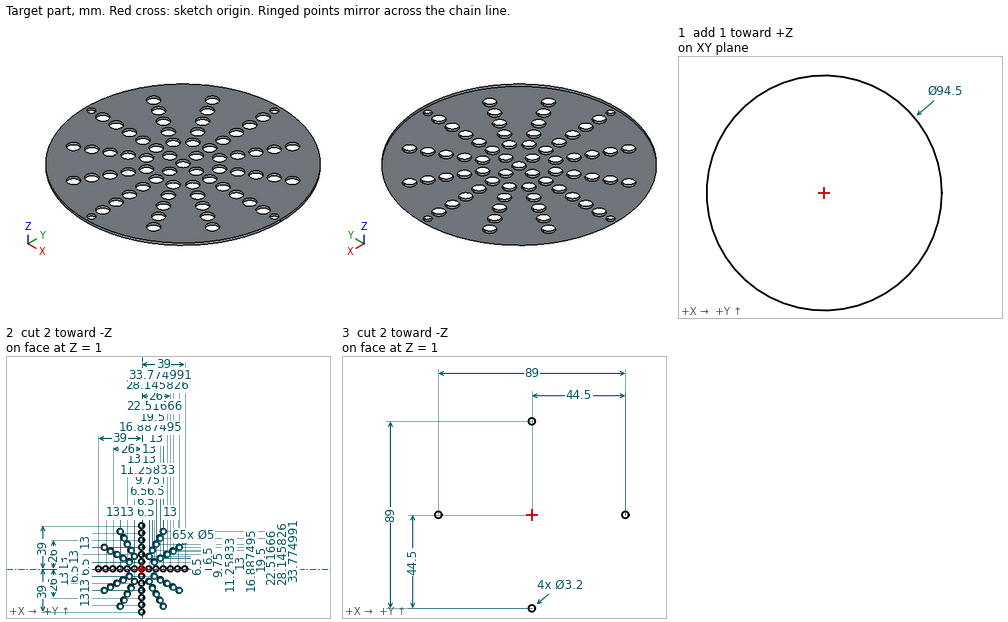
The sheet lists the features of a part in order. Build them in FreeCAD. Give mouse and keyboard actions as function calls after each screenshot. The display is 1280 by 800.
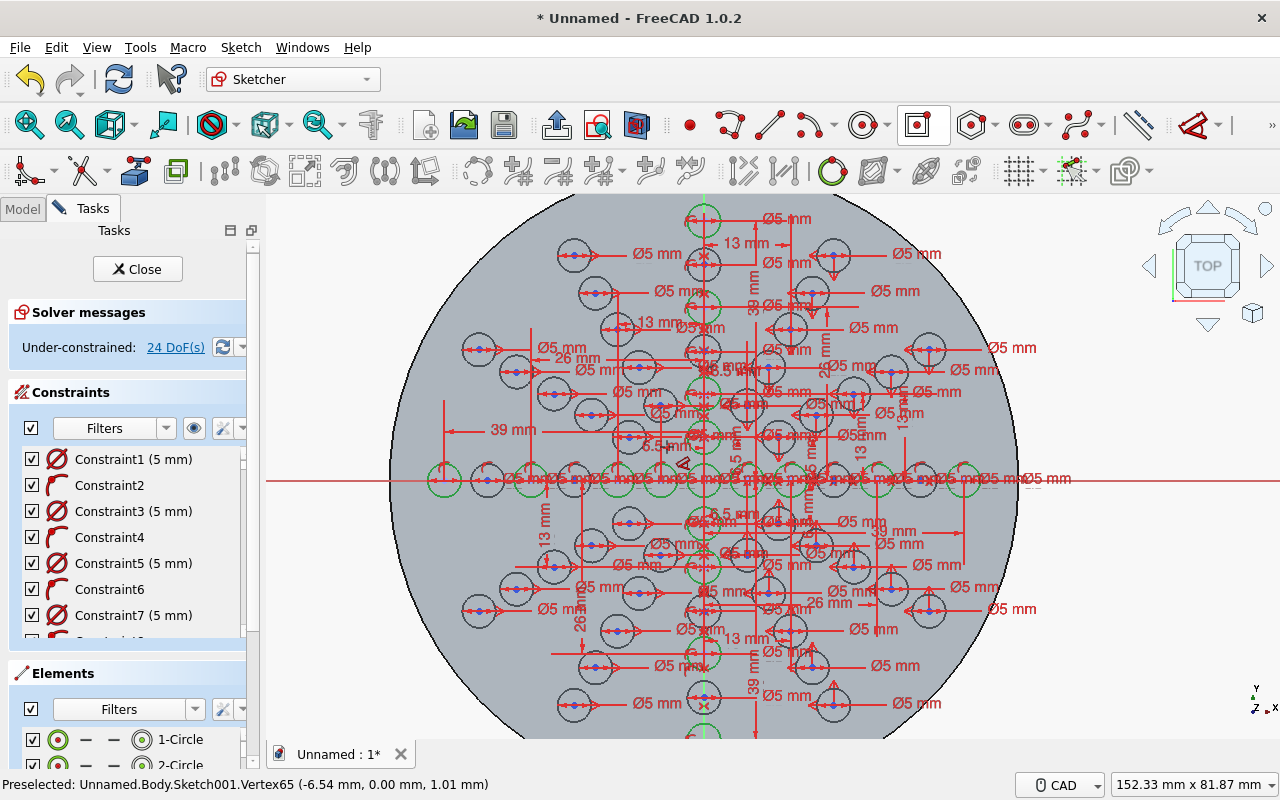
click(704, 437)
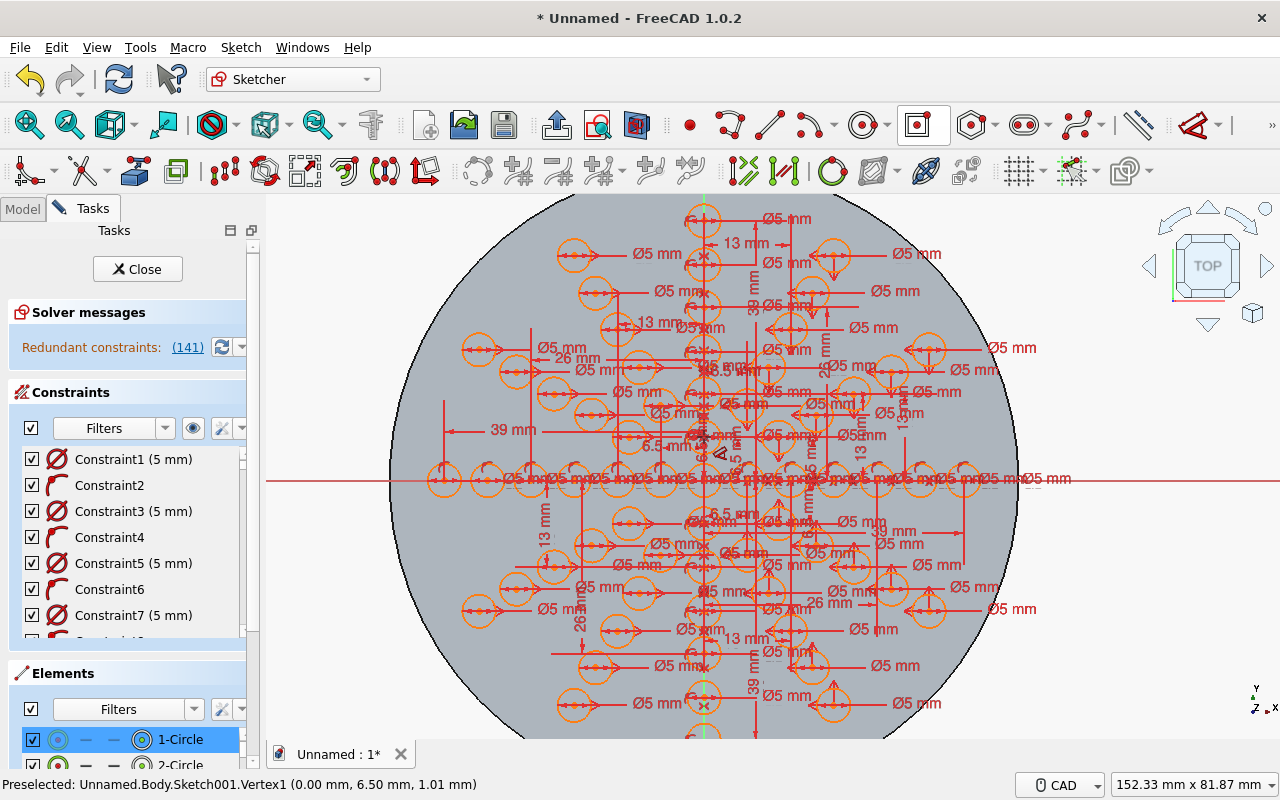
click(704, 352)
click(786, 394)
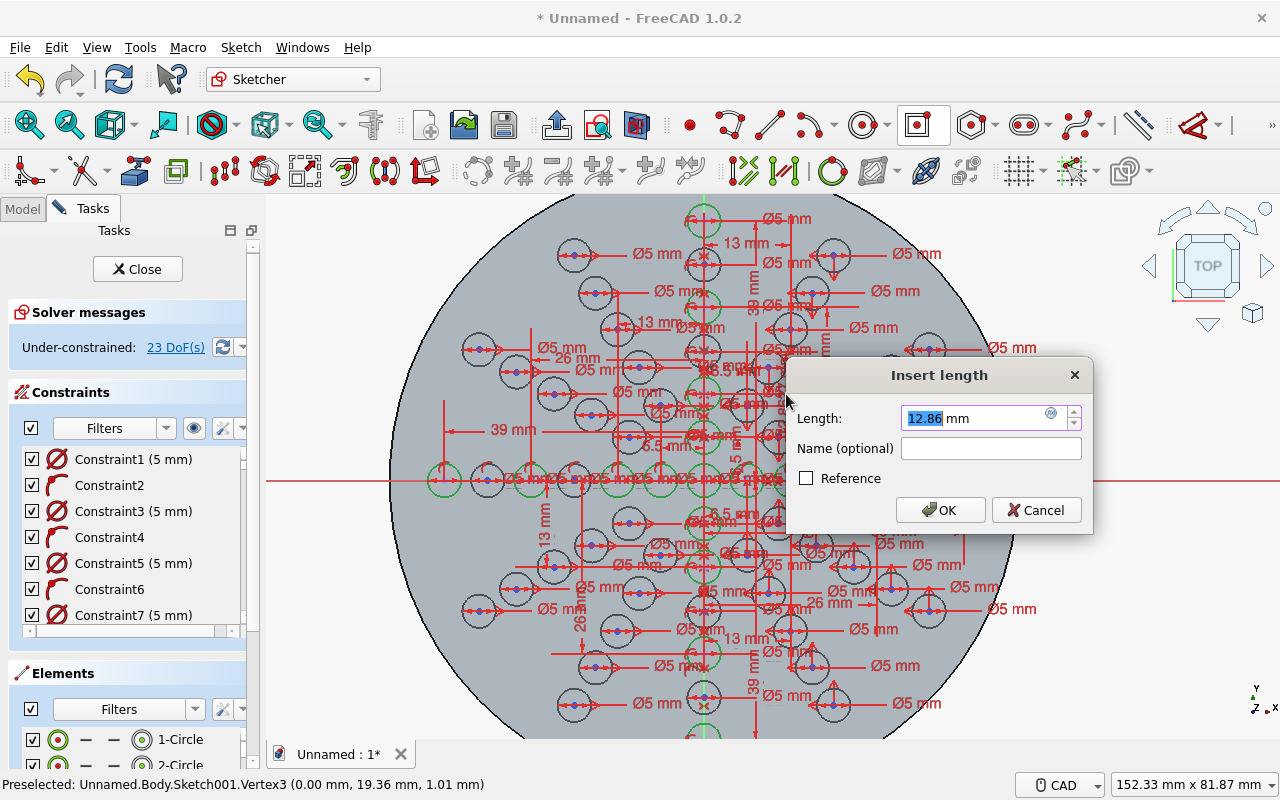
text(13)
key(Return)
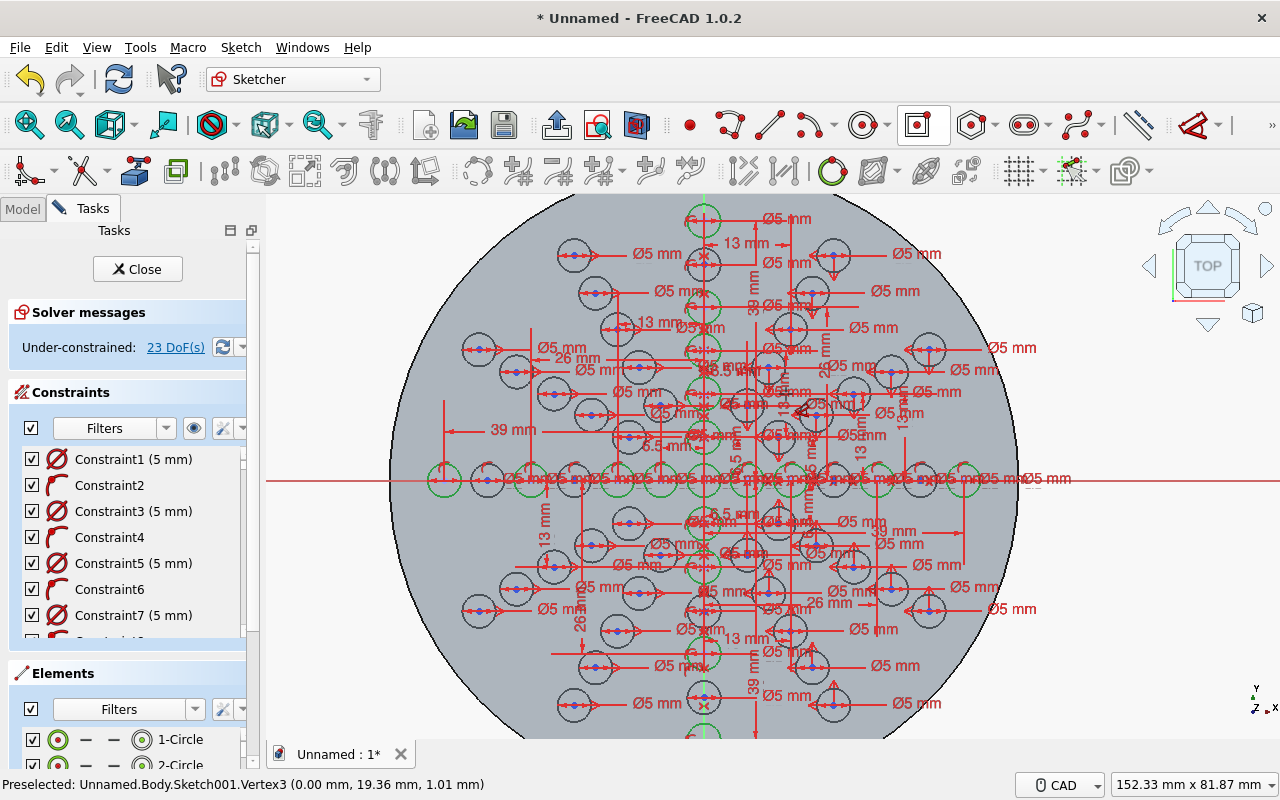
click(704, 351)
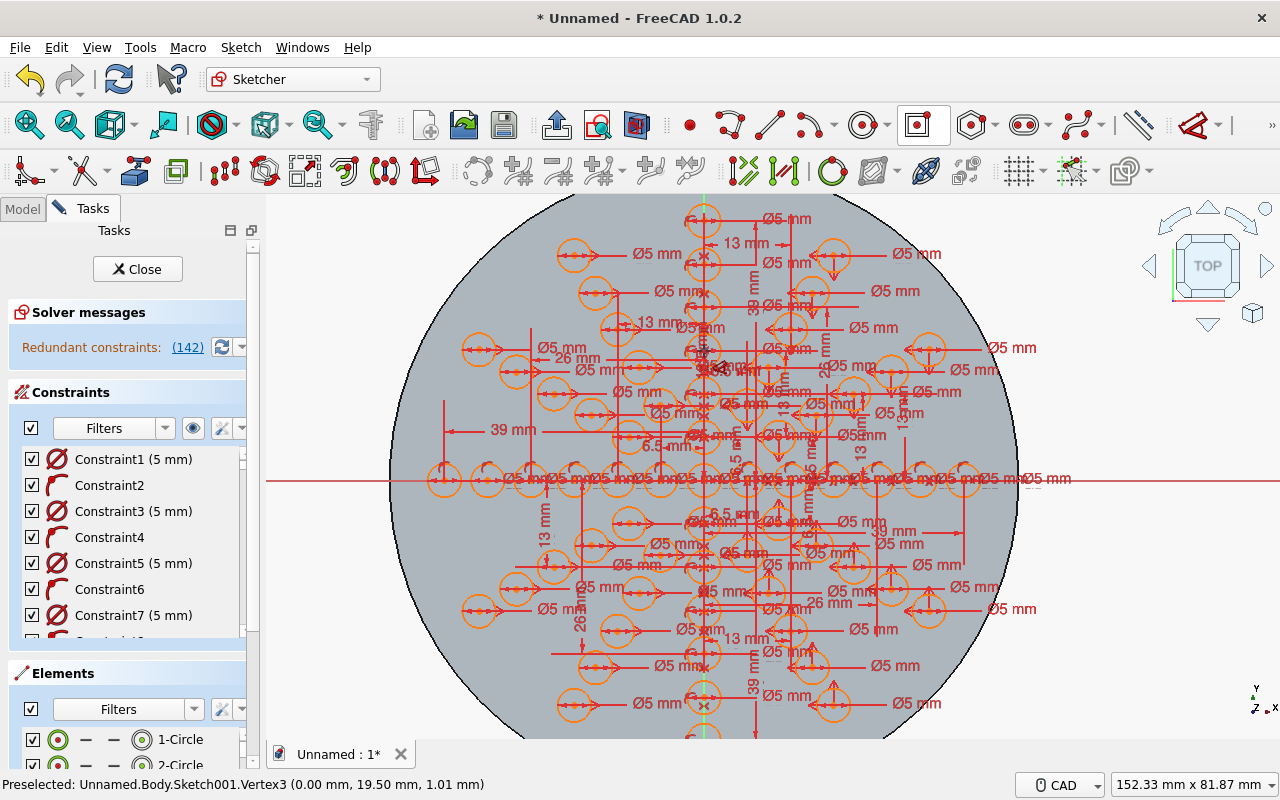
click(704, 265)
click(738, 328)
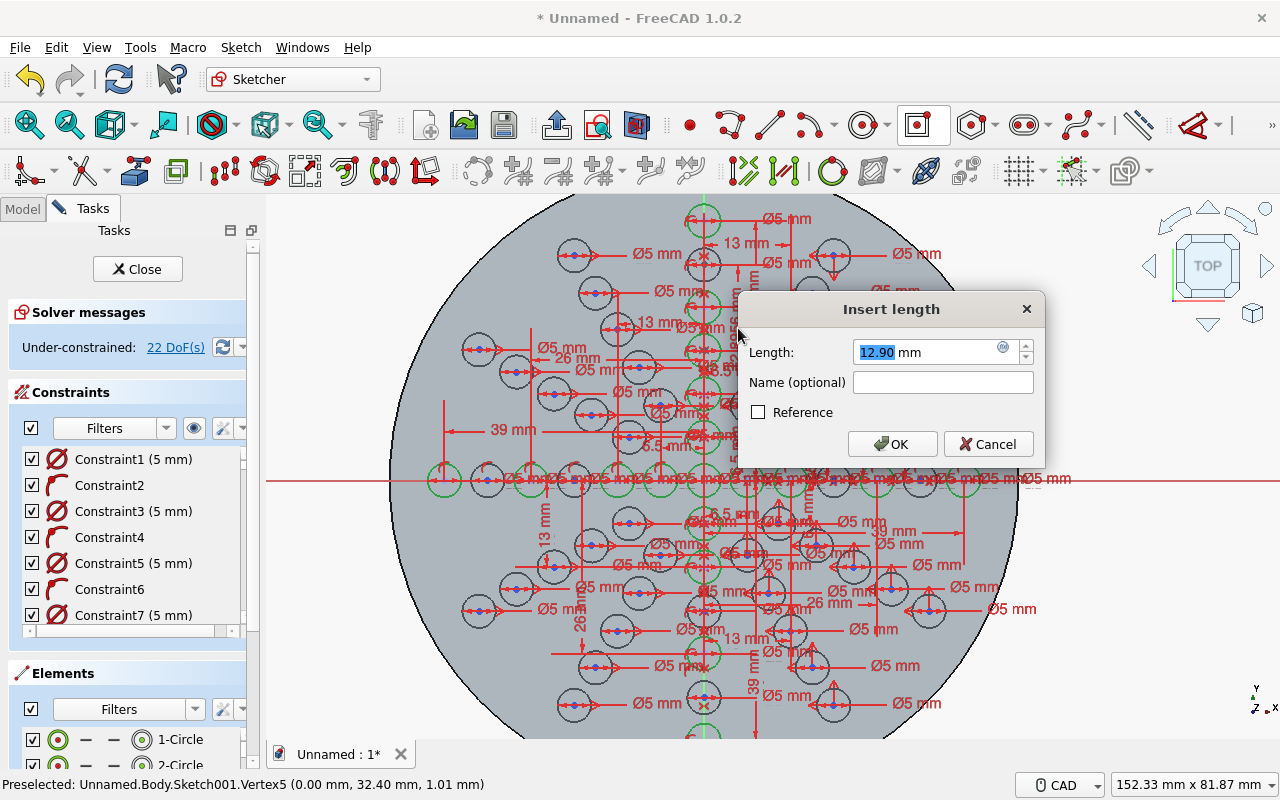
text(13)
key(Return)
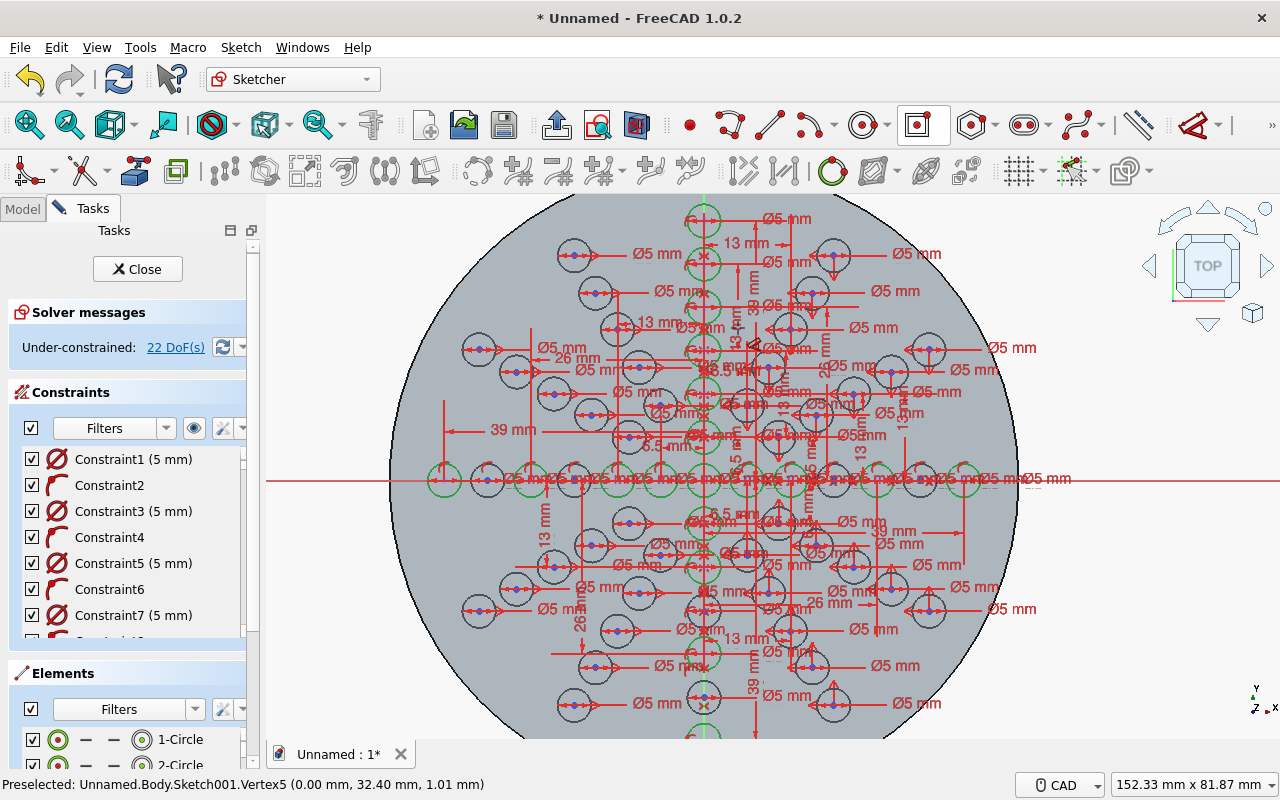
click(920, 481)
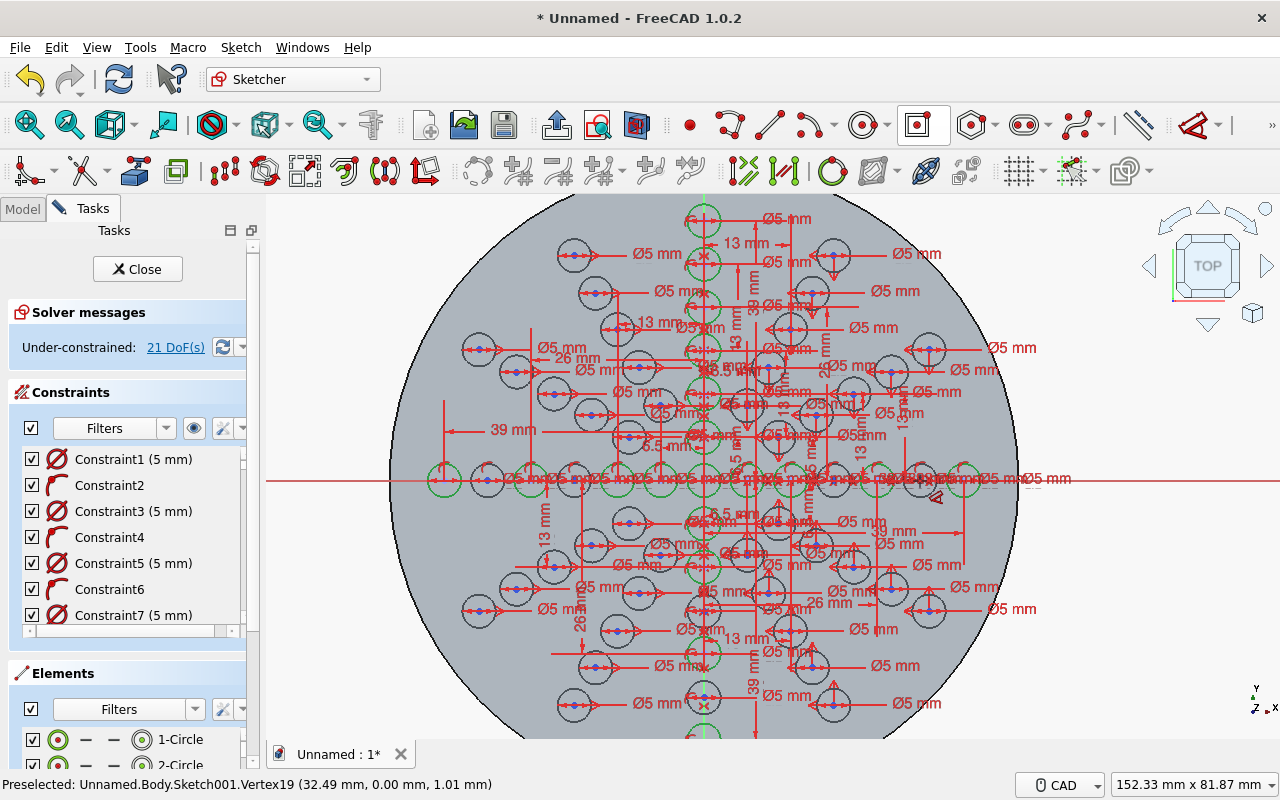
click(834, 481)
click(907, 563)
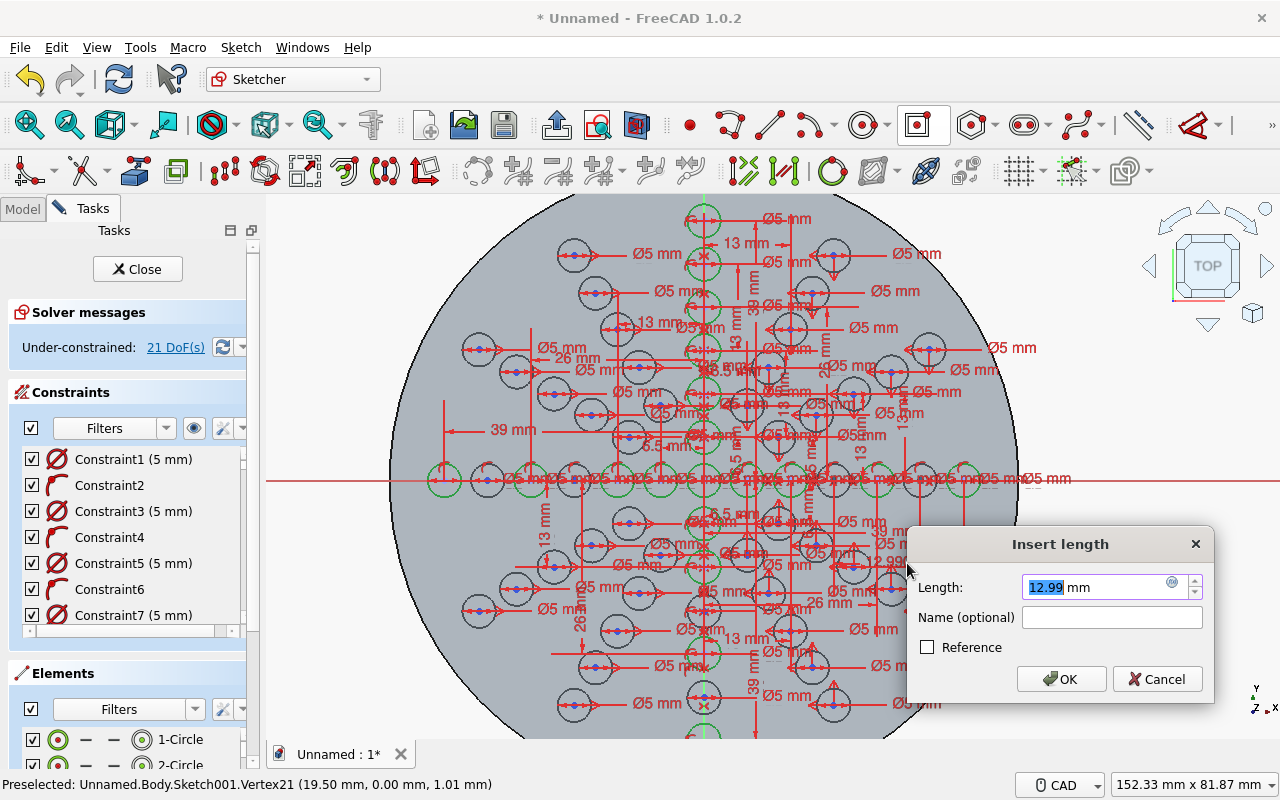
text(13)
key(Return)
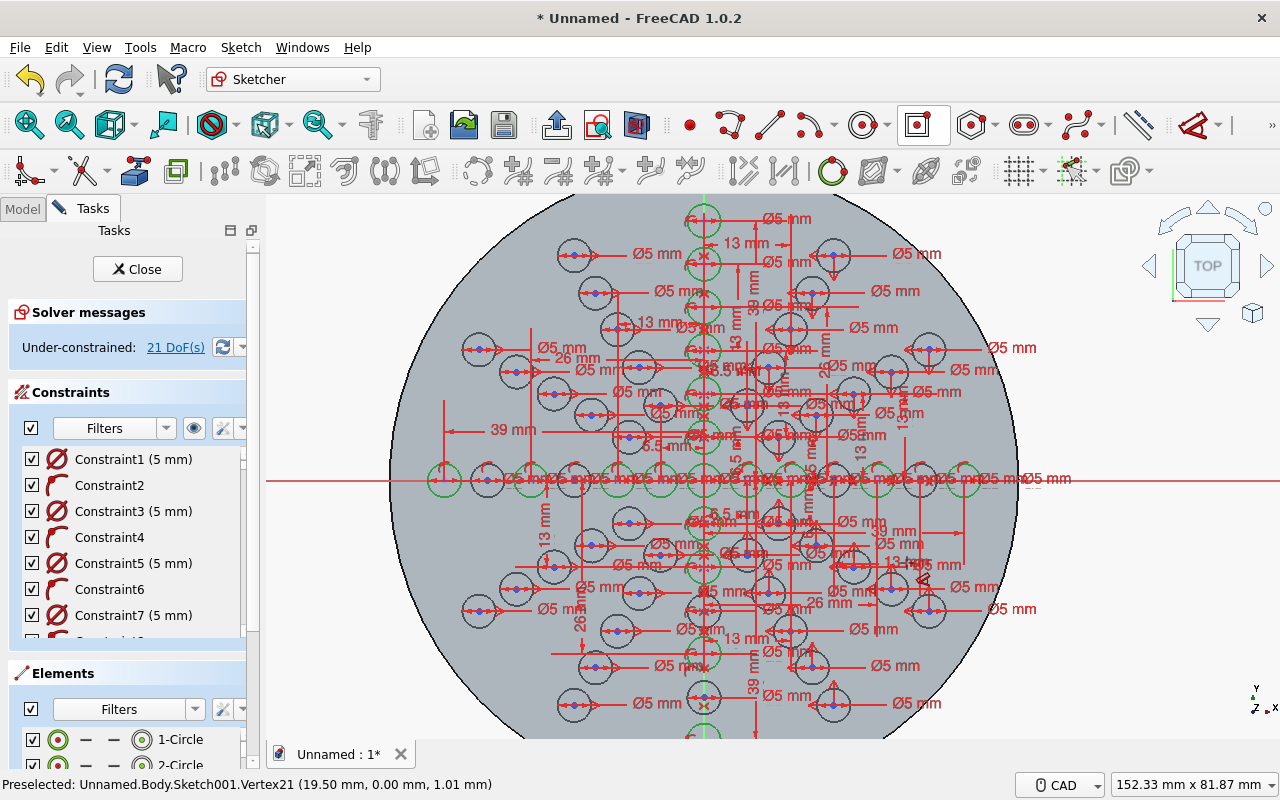
click(747, 406)